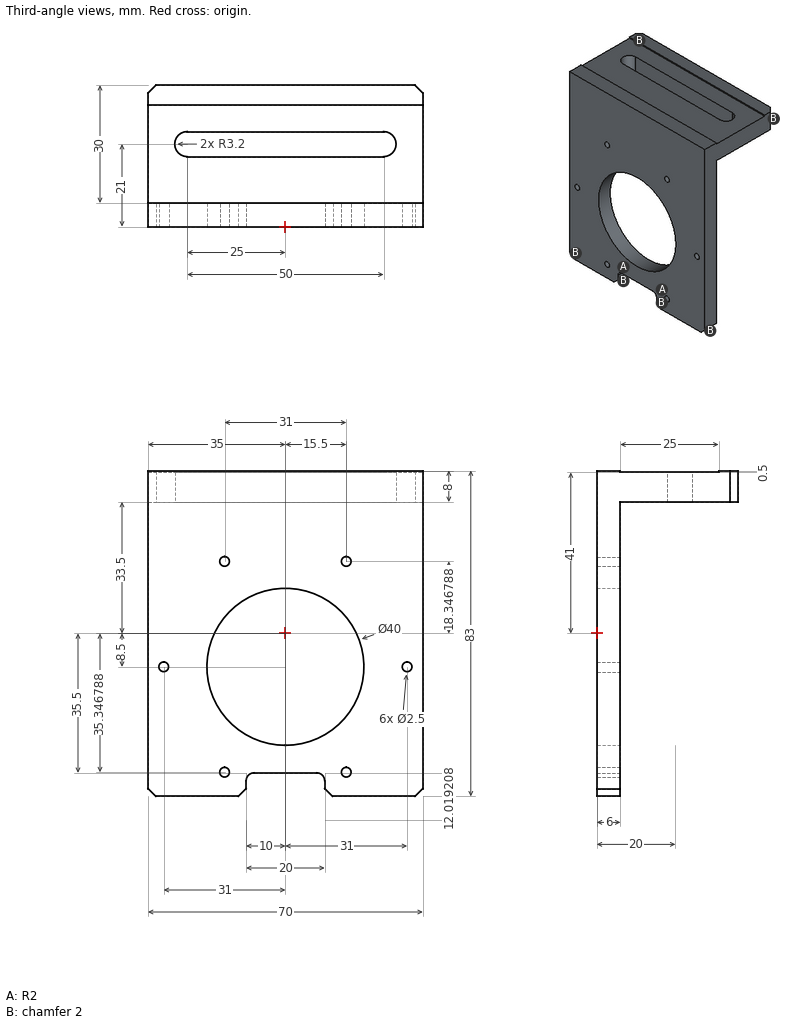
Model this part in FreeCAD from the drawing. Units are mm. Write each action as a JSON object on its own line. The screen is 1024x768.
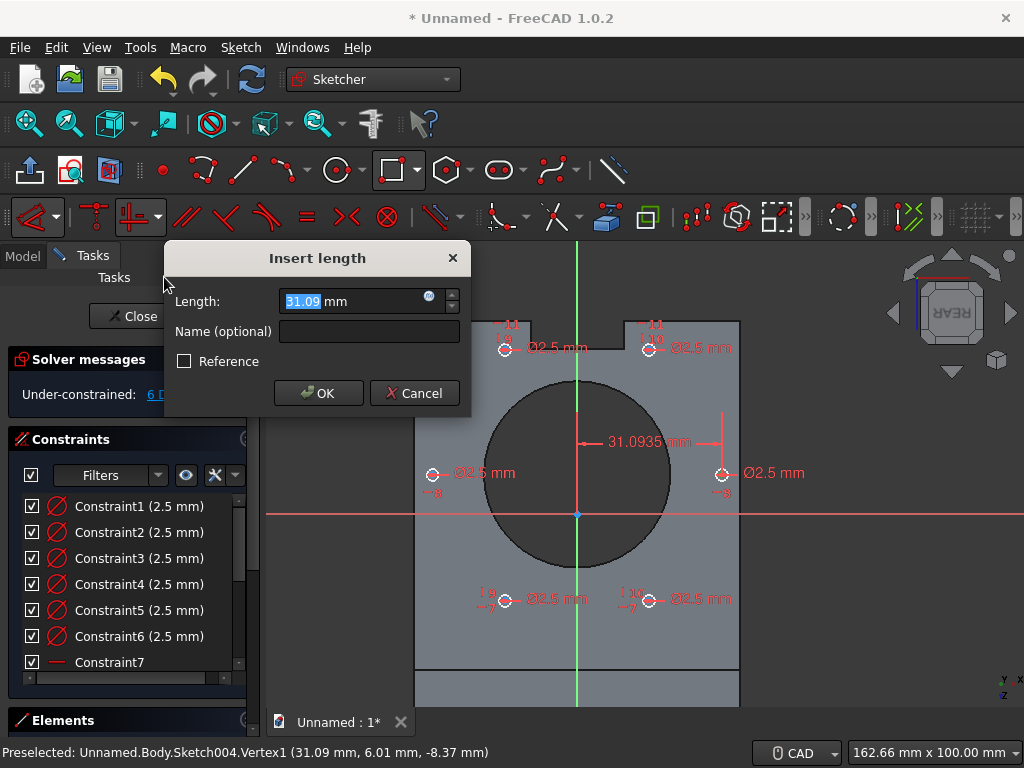
{"action": "type", "text": "31"}
{"action": "key", "text": "Return"}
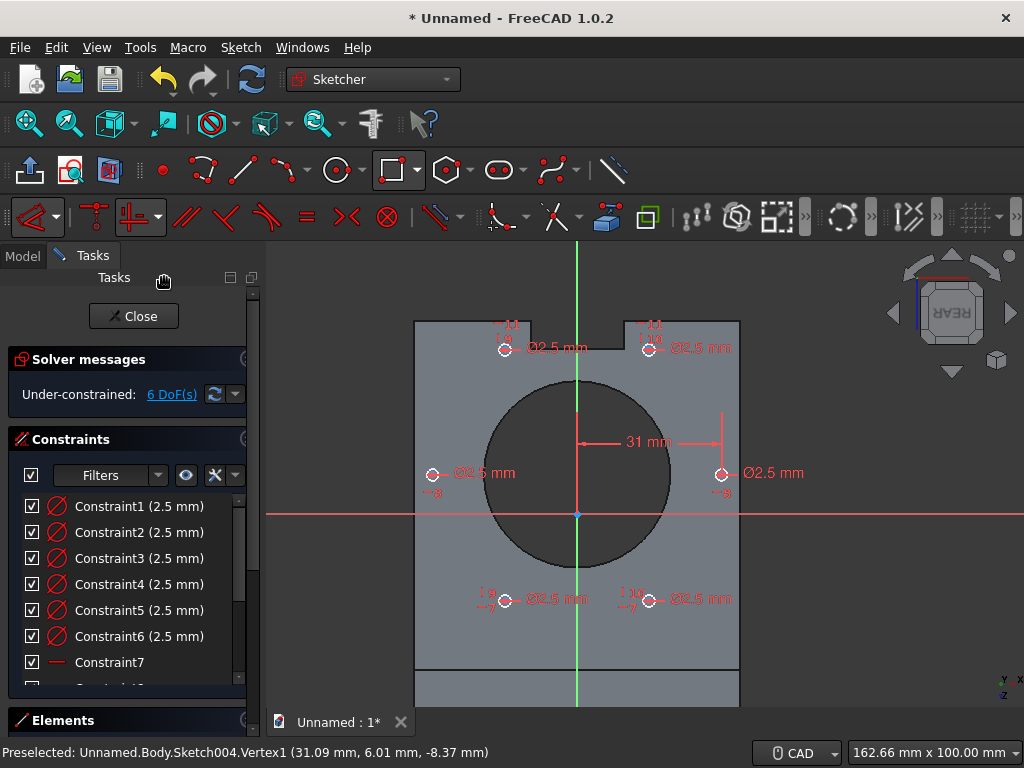
{"action": "left_click", "coordinate": [433, 475]}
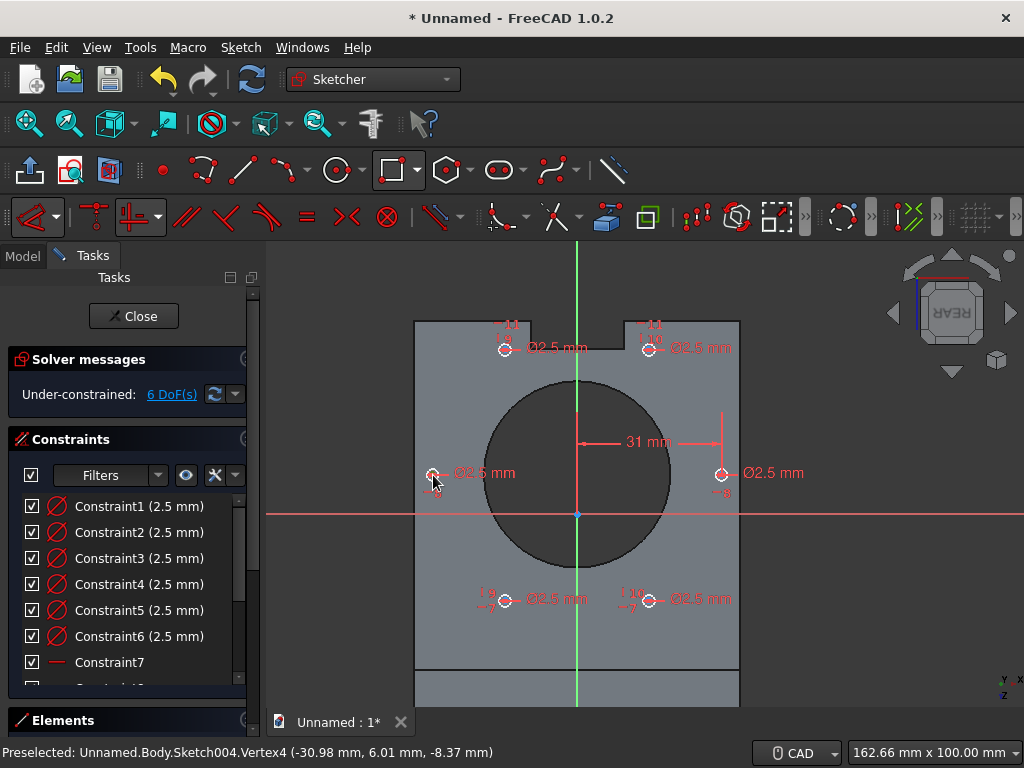
{"action": "key", "text": "l"}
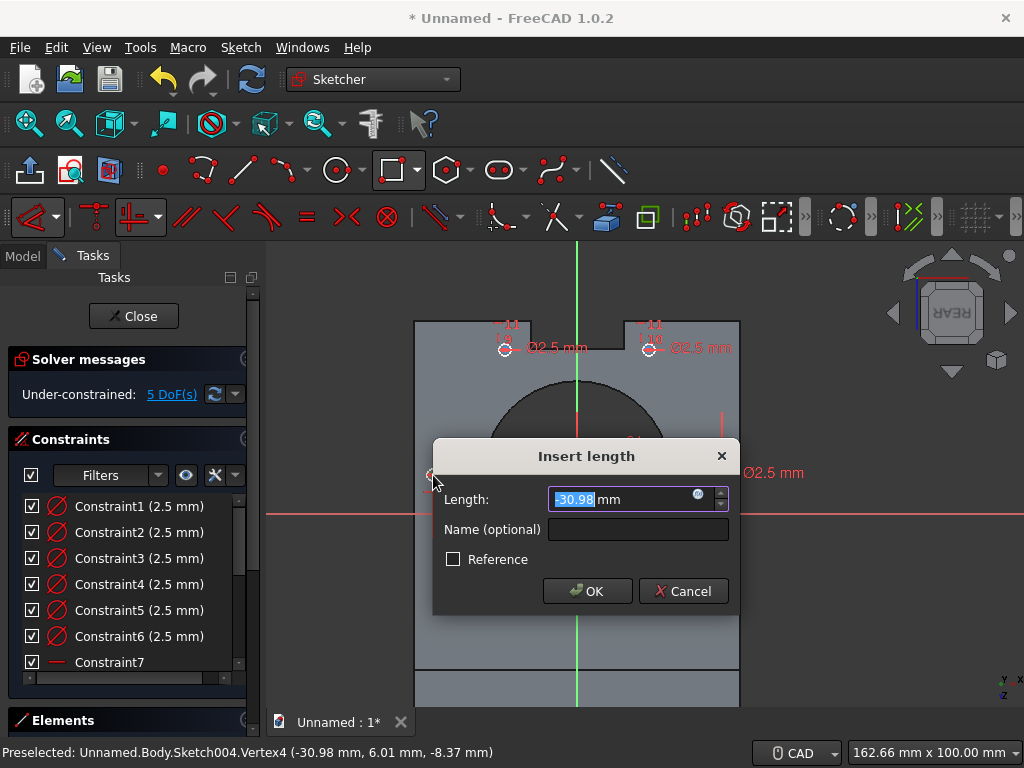
{"action": "type", "text": "-31"}
{"action": "key", "text": "Return"}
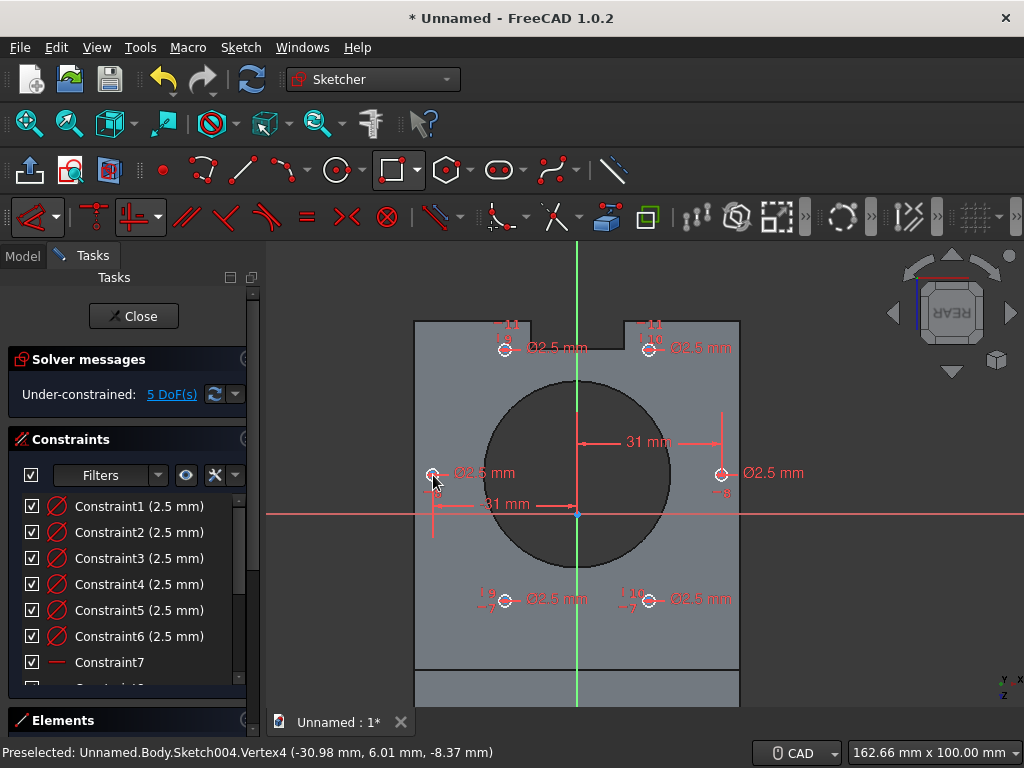
{"action": "left_click", "coordinate": [722, 475]}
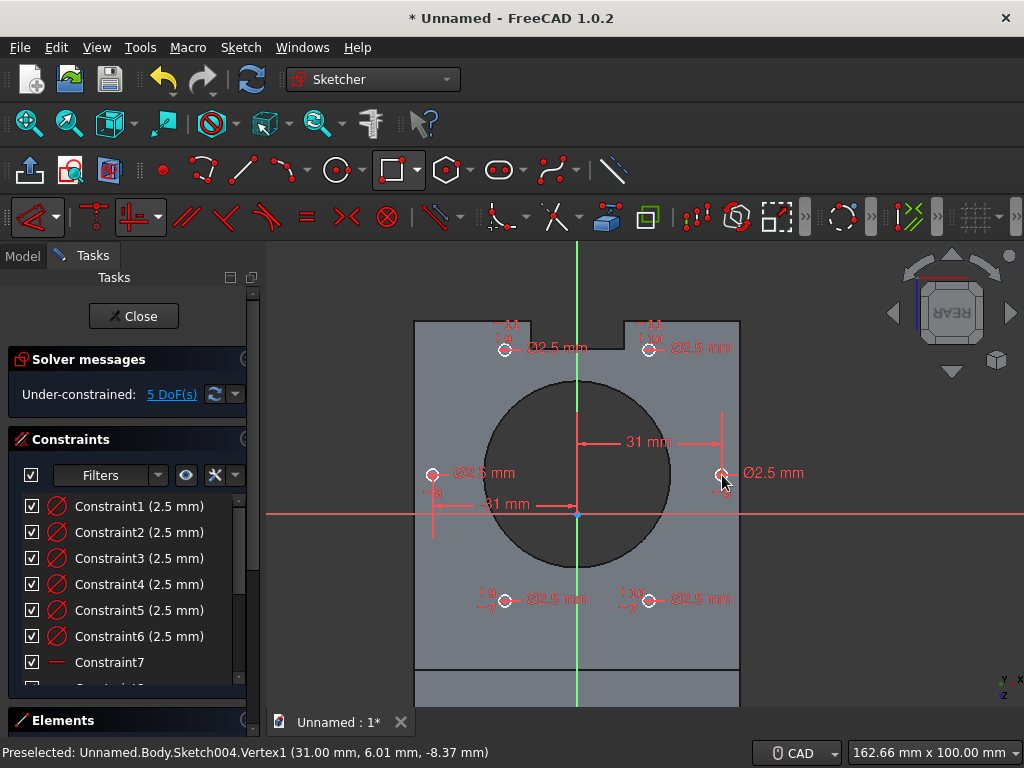
{"action": "key", "text": "i"}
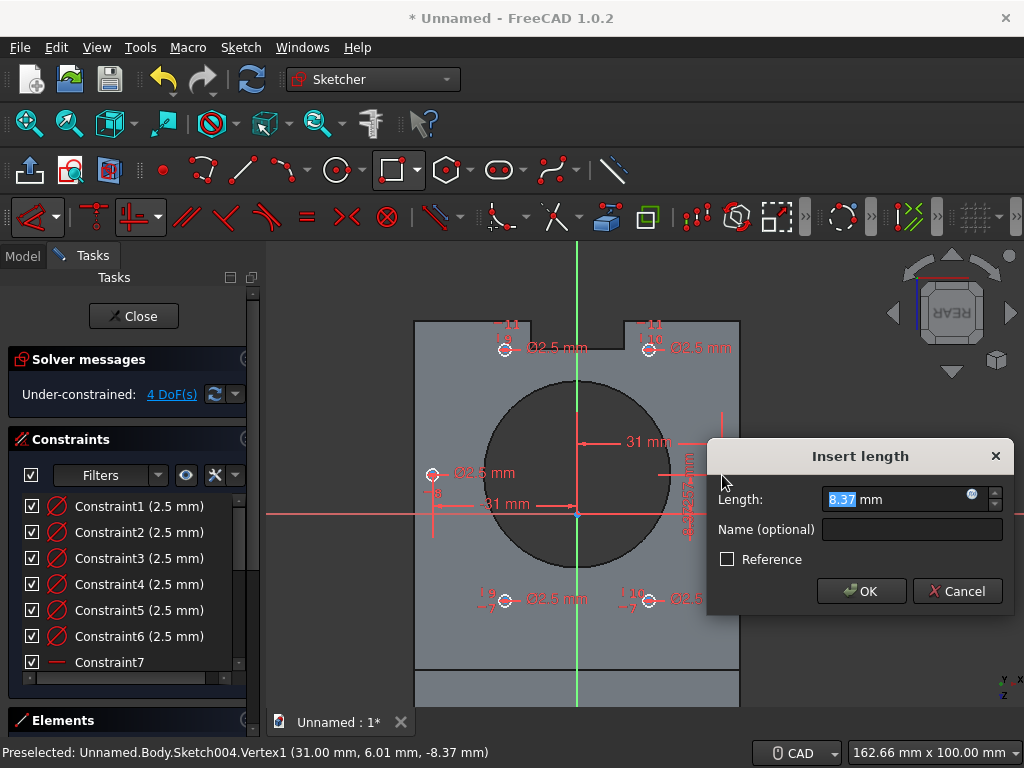
{"action": "type", "text": "8.5"}
{"action": "key", "text": "Return"}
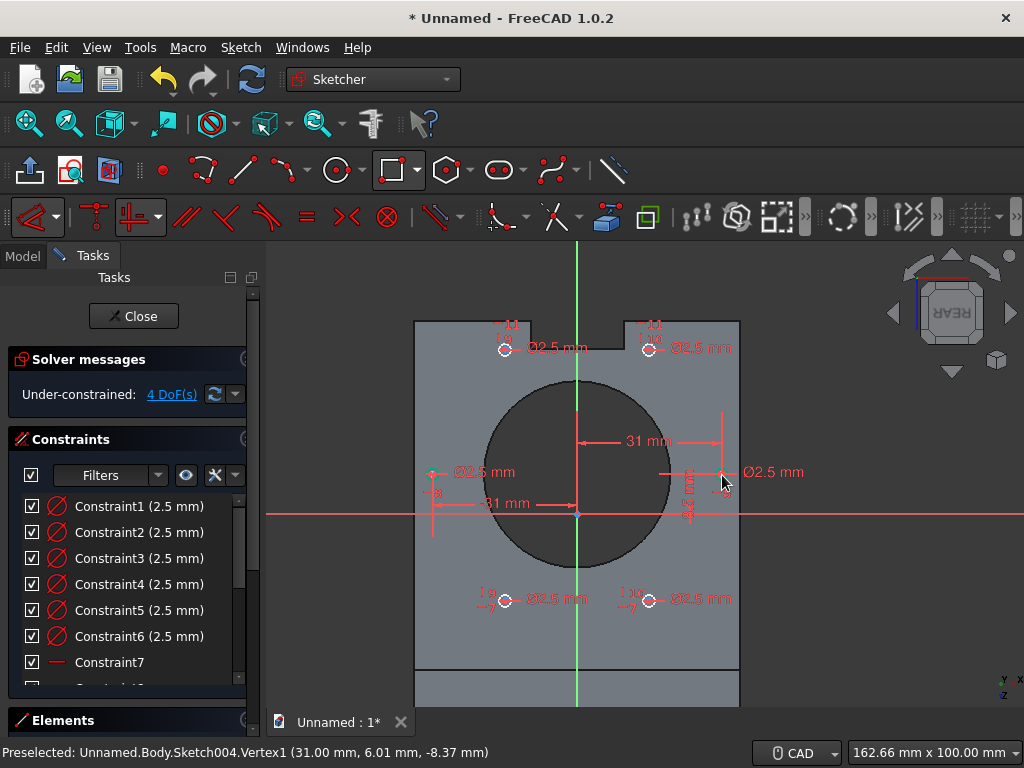
{"action": "left_click", "coordinate": [649, 601]}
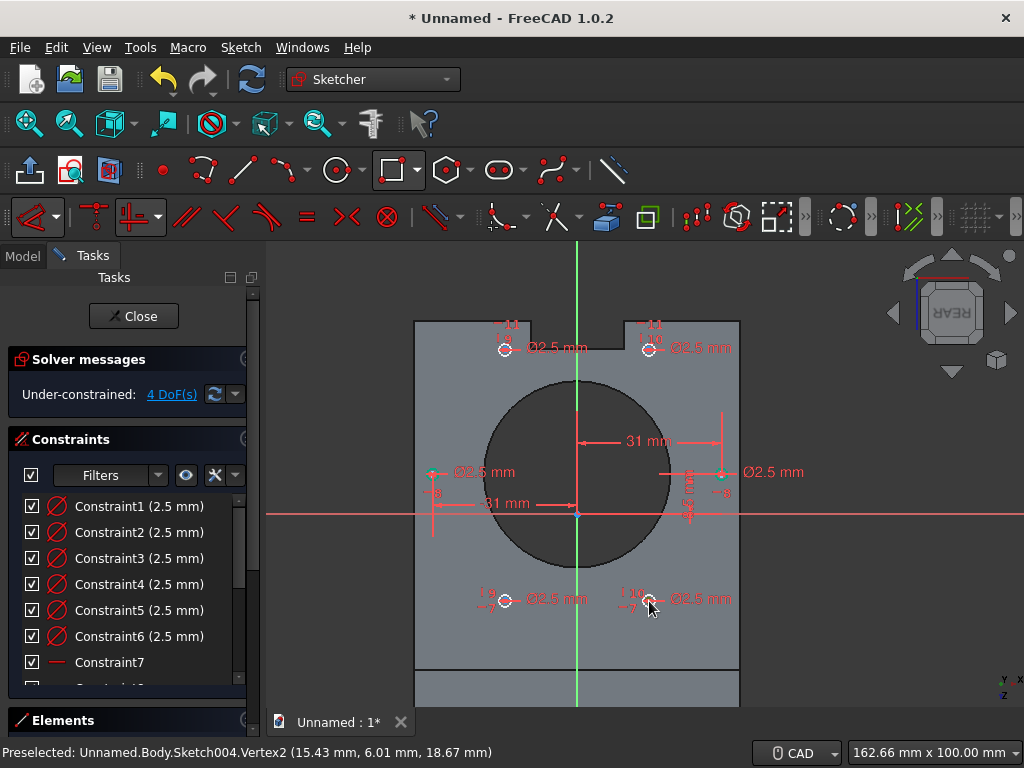
{"action": "left_click", "coordinate": [505, 601]}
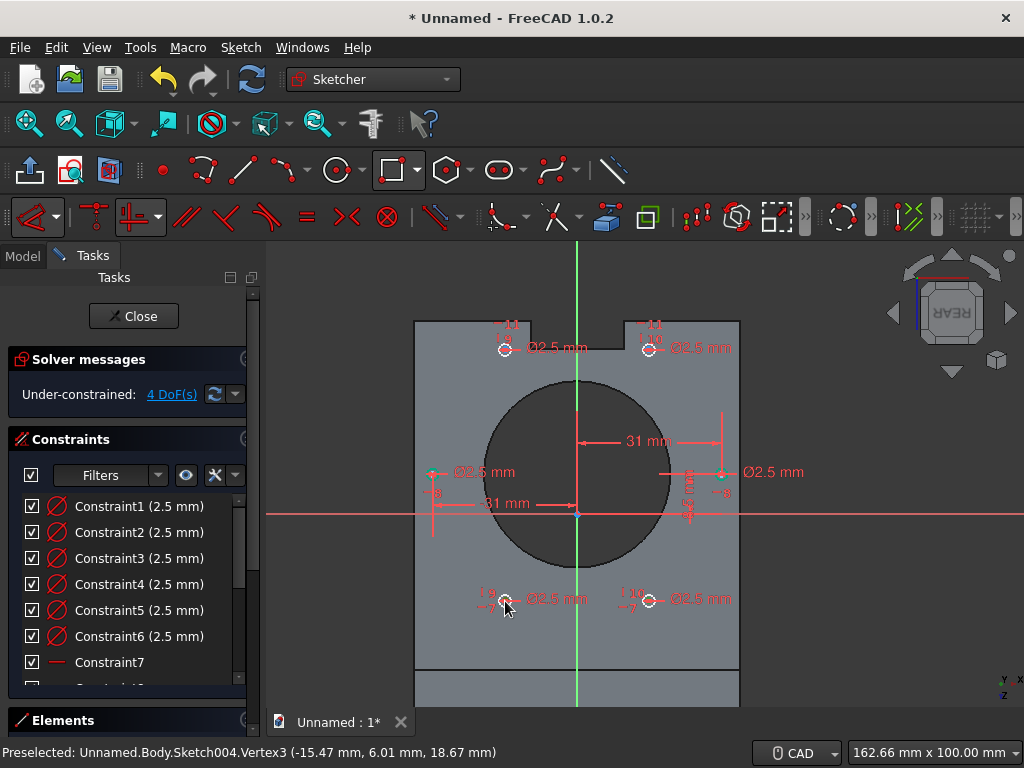
{"action": "key", "text": "l"}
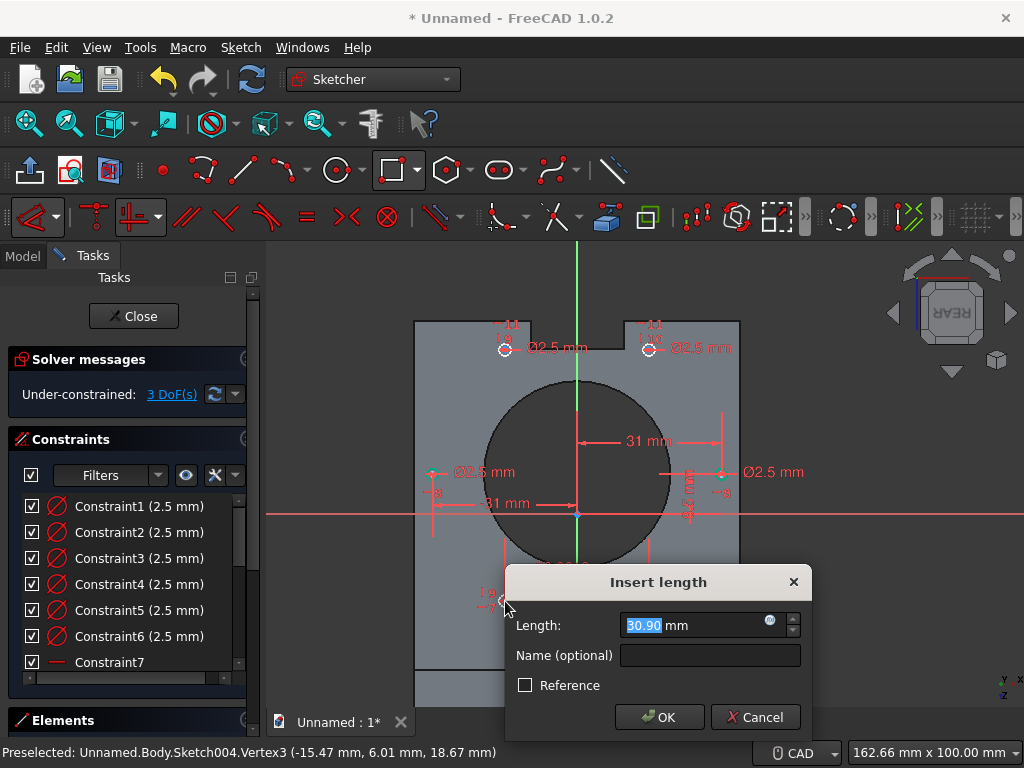
{"action": "type", "text": "31"}
{"action": "key", "text": "Return"}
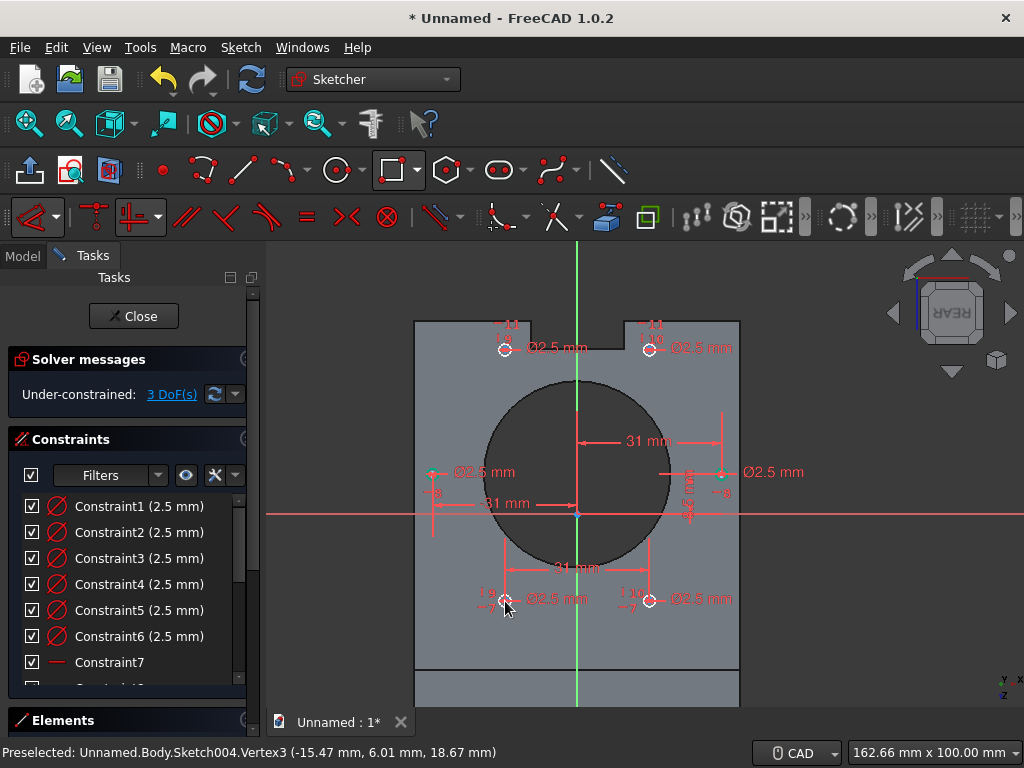
{"action": "left_click", "coordinate": [649, 601]}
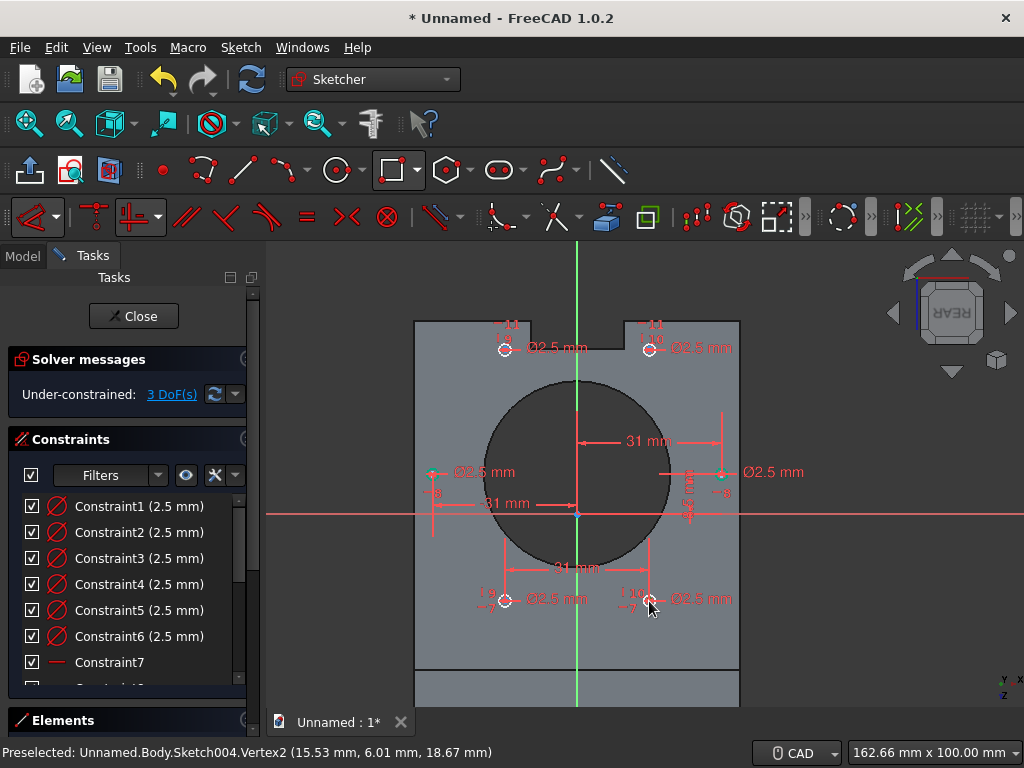
{"action": "left_click", "coordinate": [58, 218]}